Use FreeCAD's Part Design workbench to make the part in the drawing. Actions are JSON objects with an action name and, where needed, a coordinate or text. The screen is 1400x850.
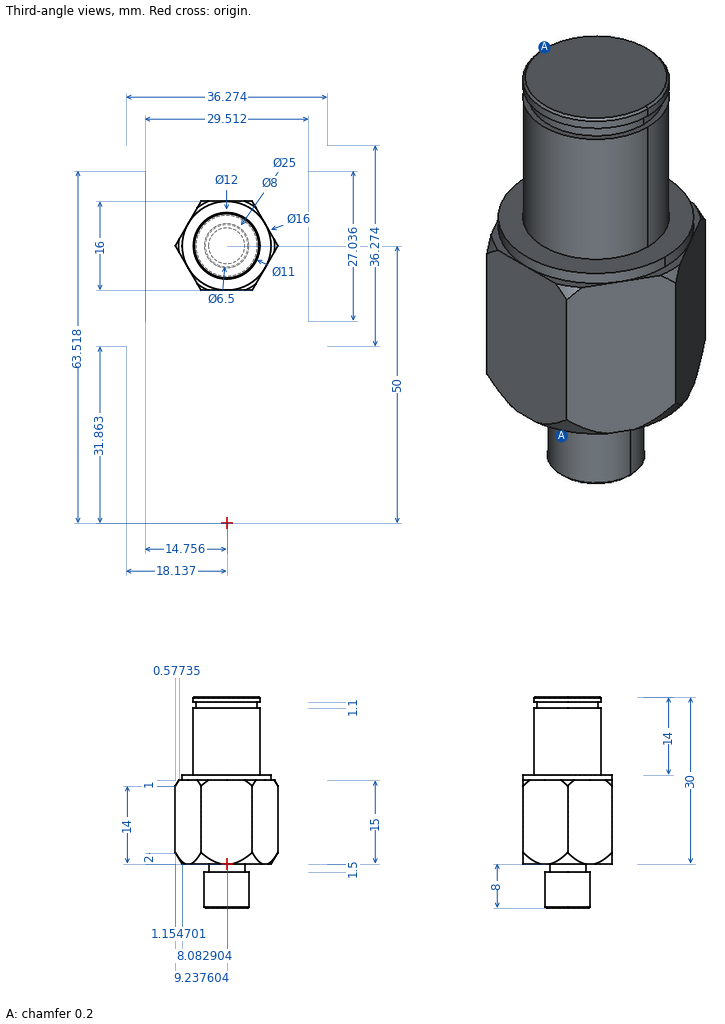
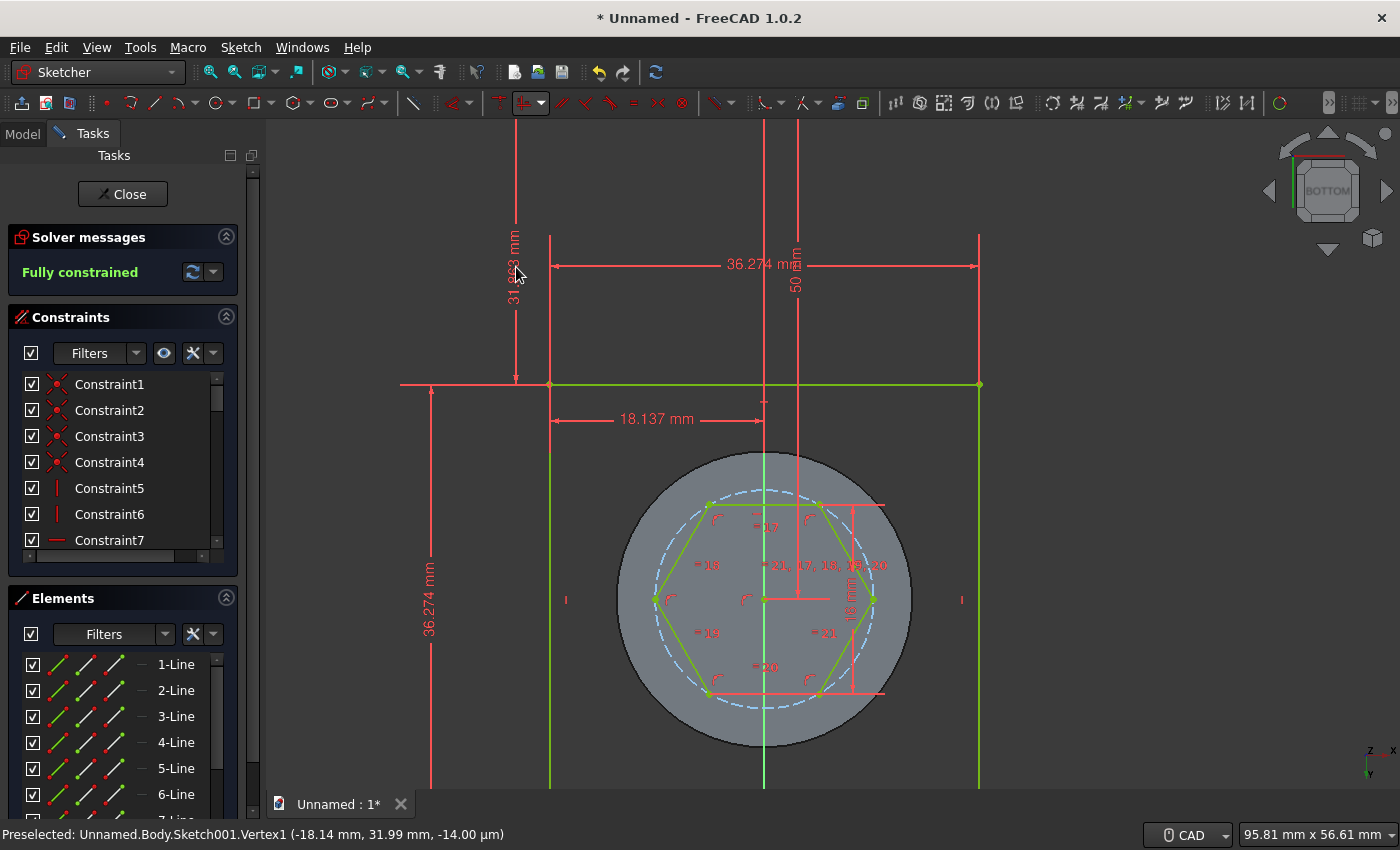
{"action": "left_click", "coordinate": [123, 194]}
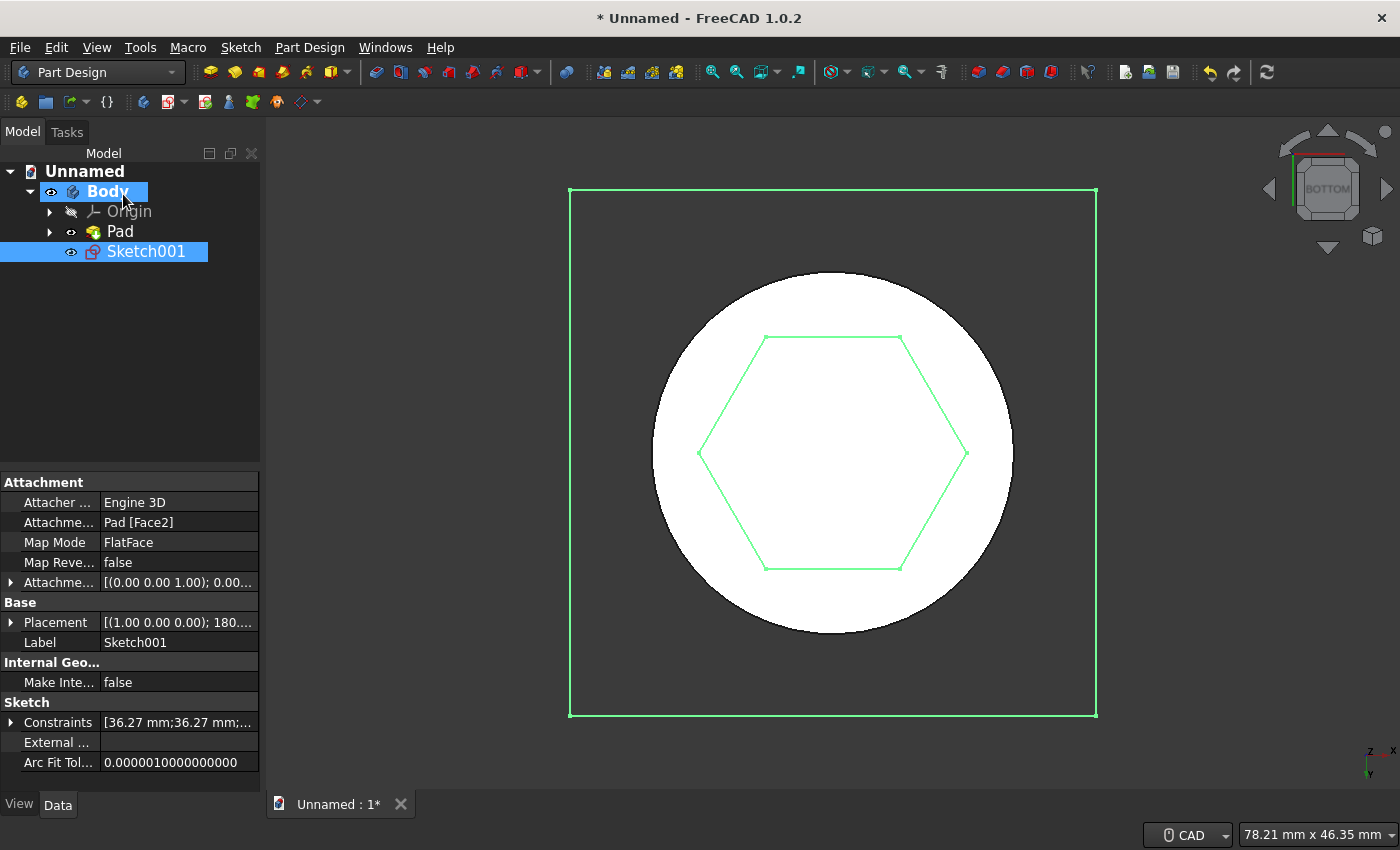
{"action": "left_click", "coordinate": [378, 72]}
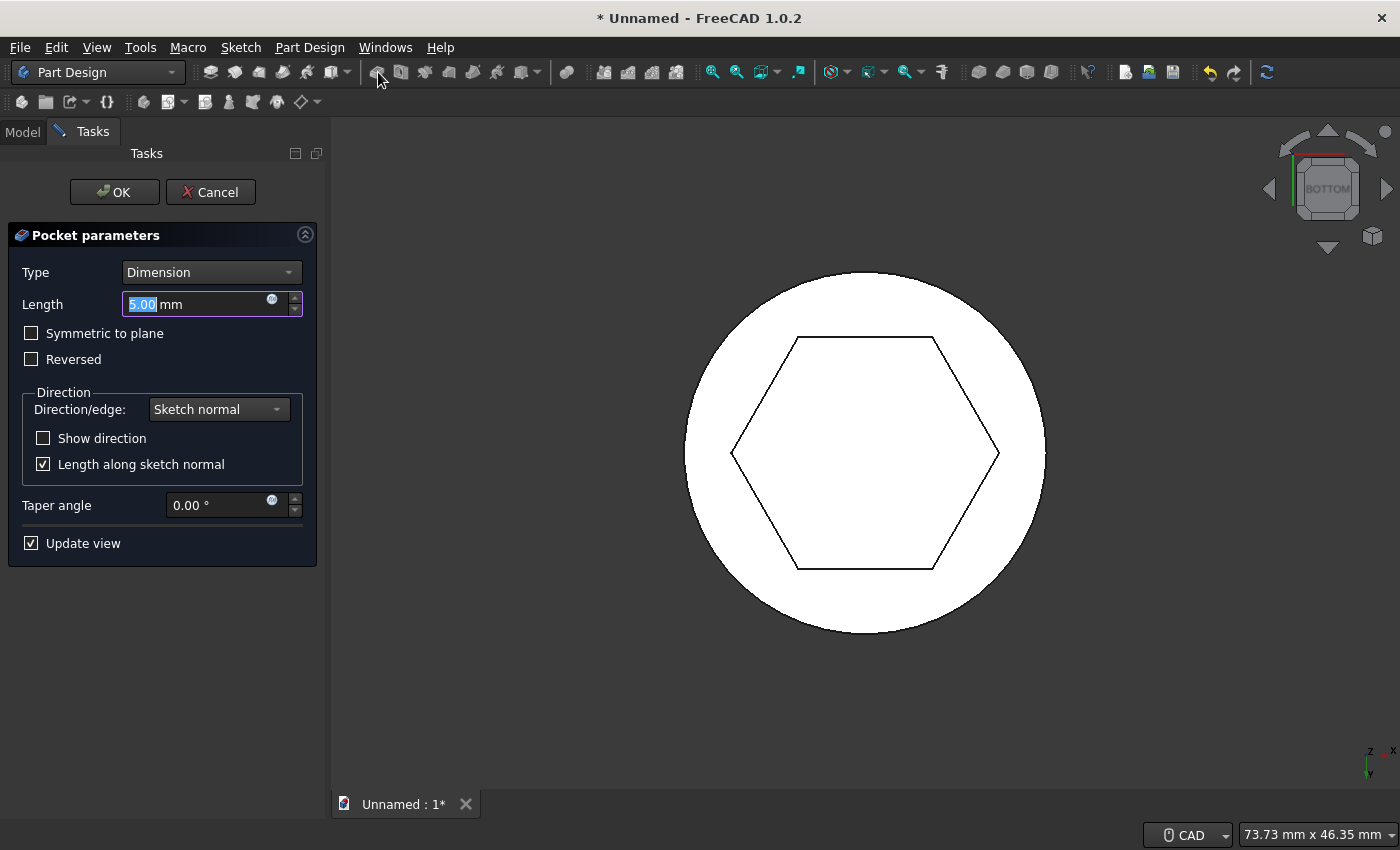
{"action": "type", "text": "15"}
{"action": "key", "text": "Tab"}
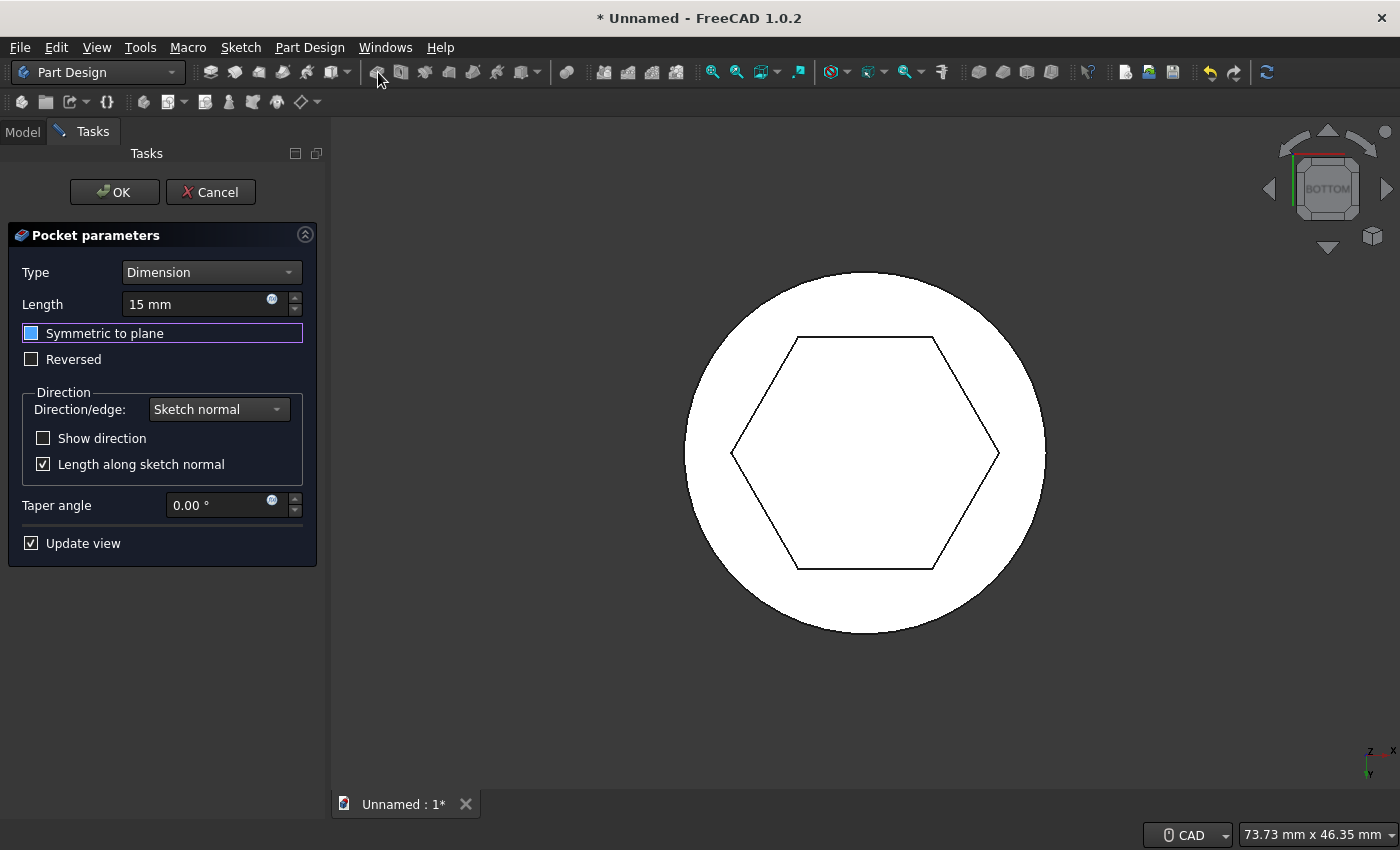
{"action": "left_click", "coordinate": [115, 192]}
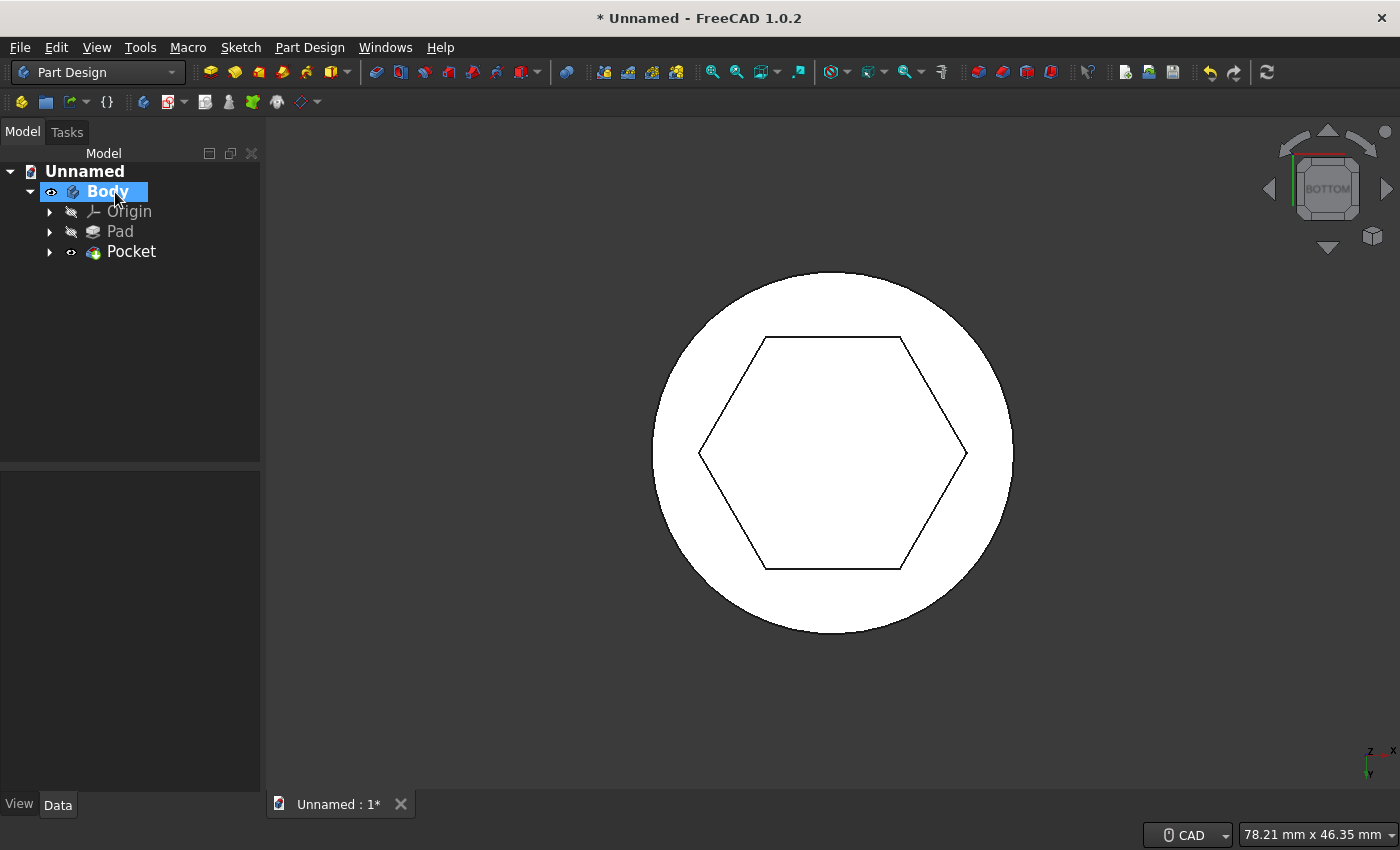
{"action": "left_click", "coordinate": [833, 607]}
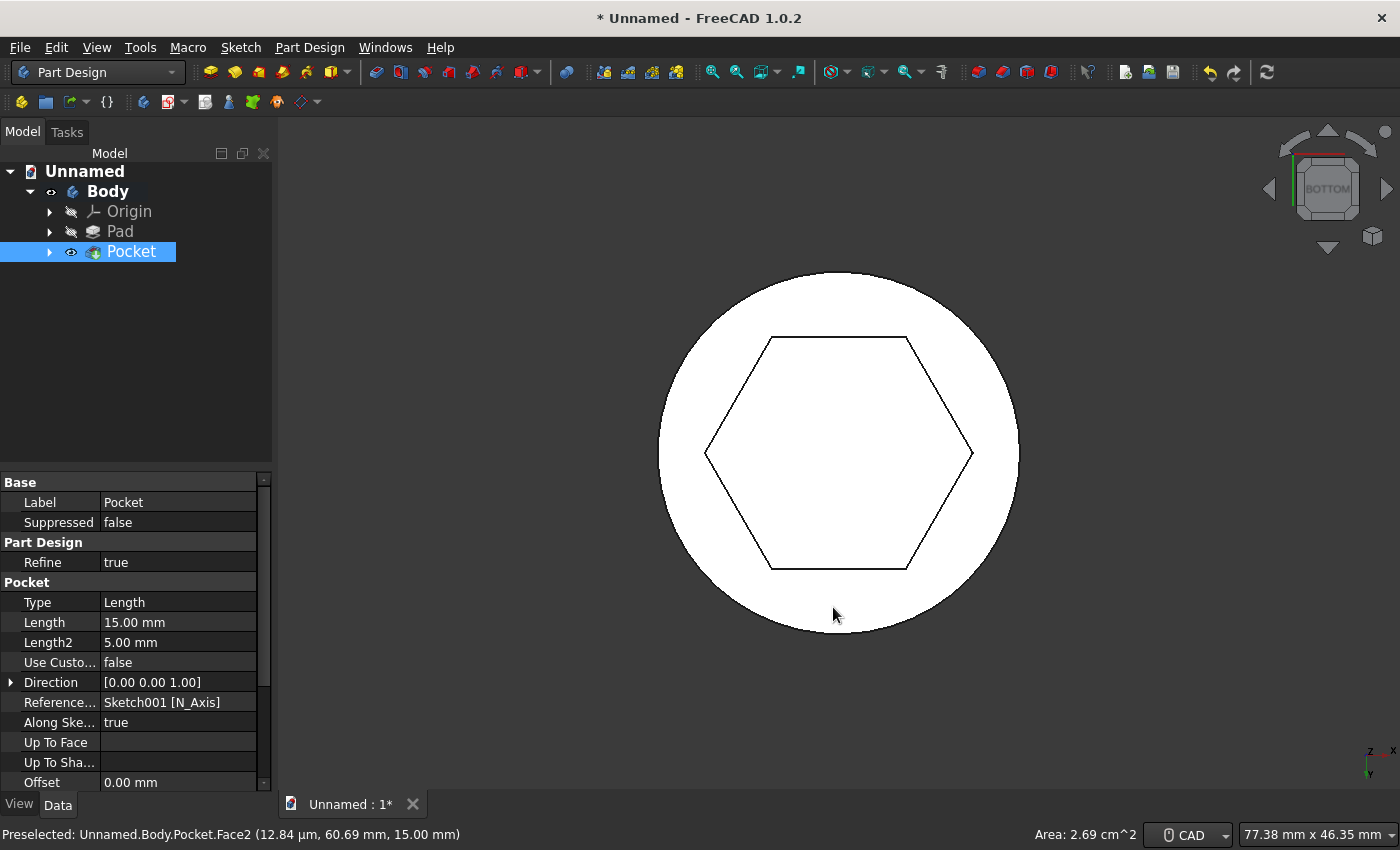
{"action": "left_click", "coordinate": [168, 102]}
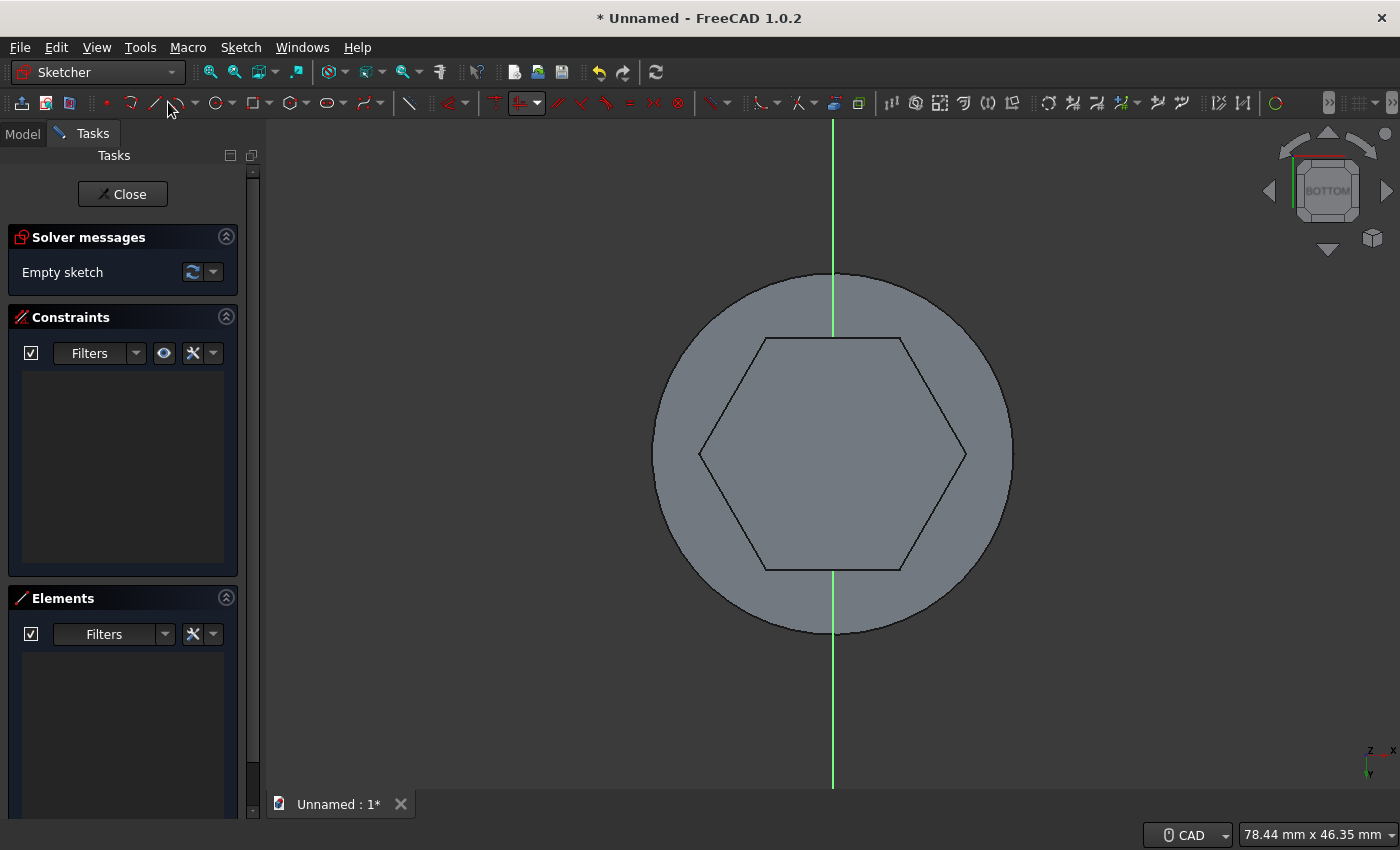
{"action": "scroll", "coordinate": [709, 642], "scroll_direction": "down", "scroll_amount": 4}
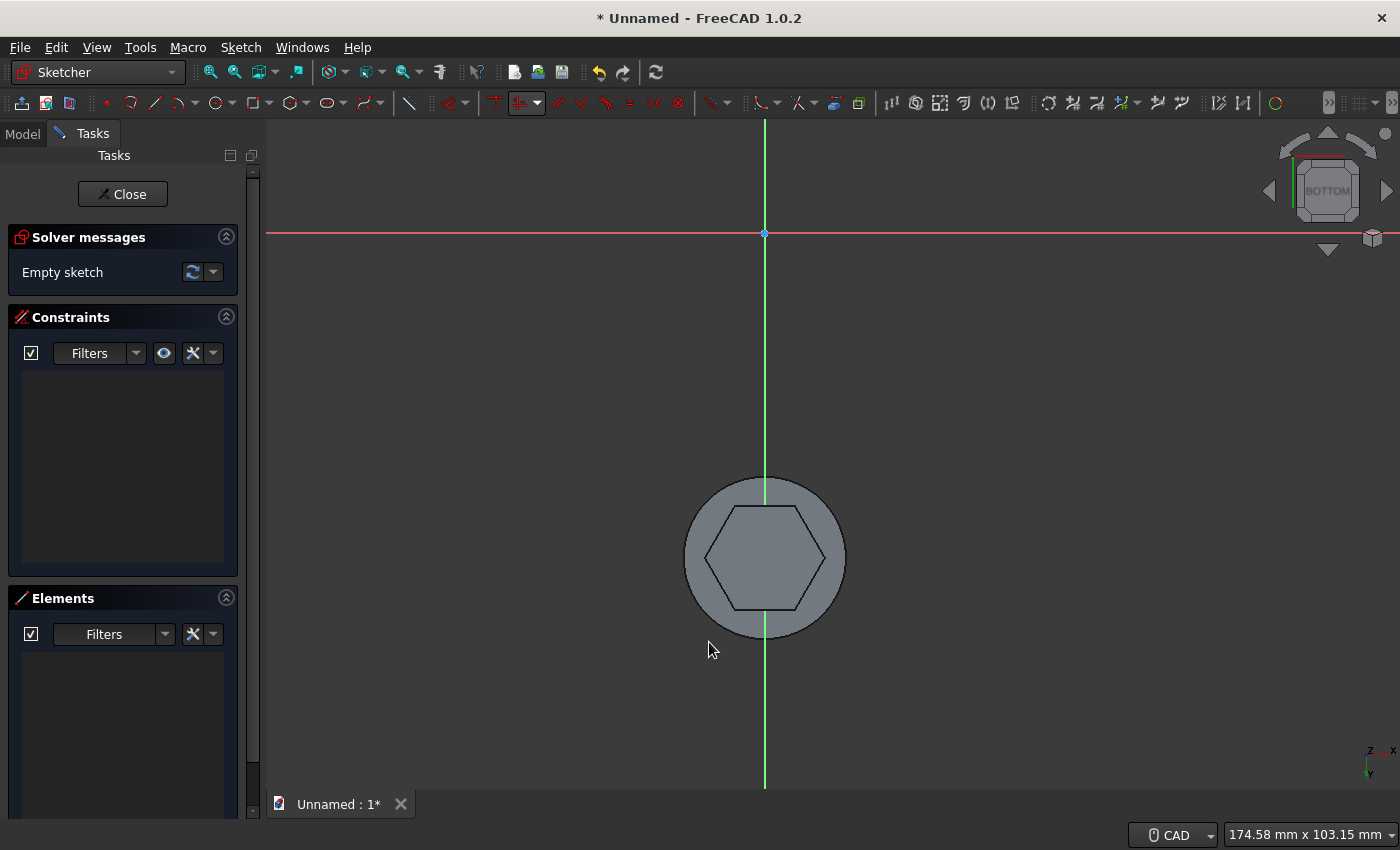
{"action": "left_click", "coordinate": [254, 104]}